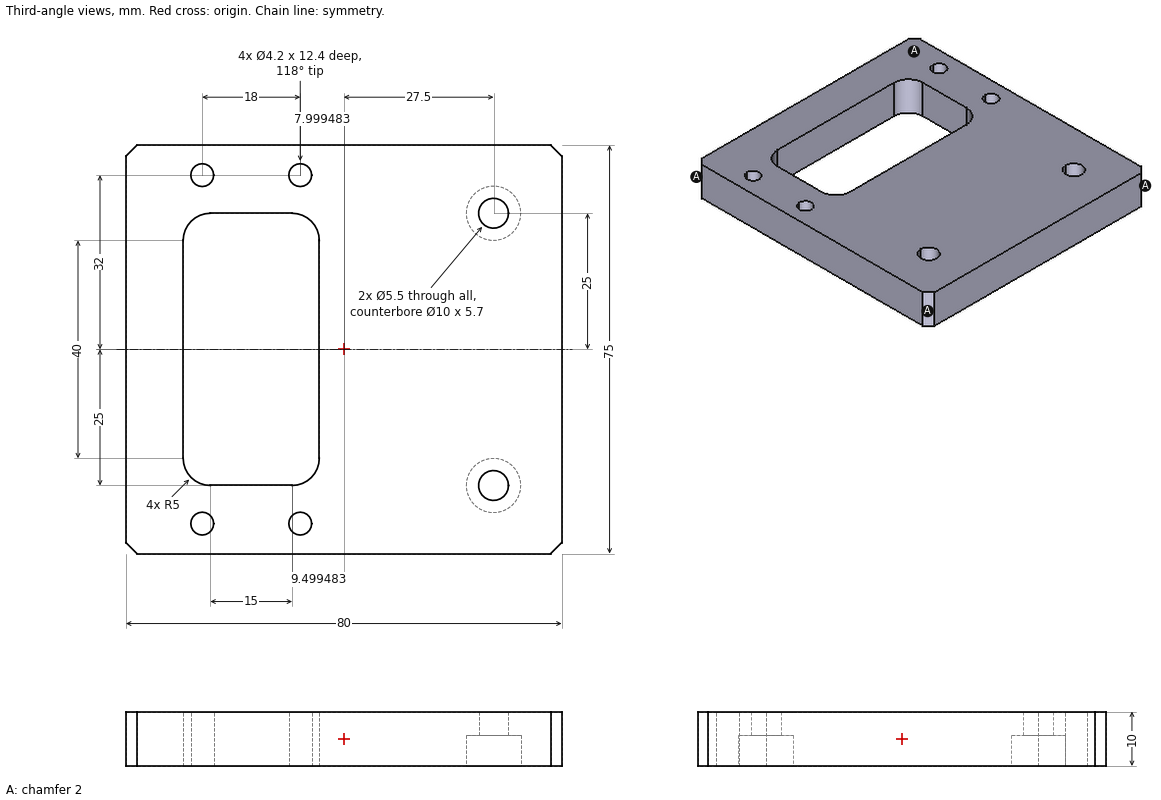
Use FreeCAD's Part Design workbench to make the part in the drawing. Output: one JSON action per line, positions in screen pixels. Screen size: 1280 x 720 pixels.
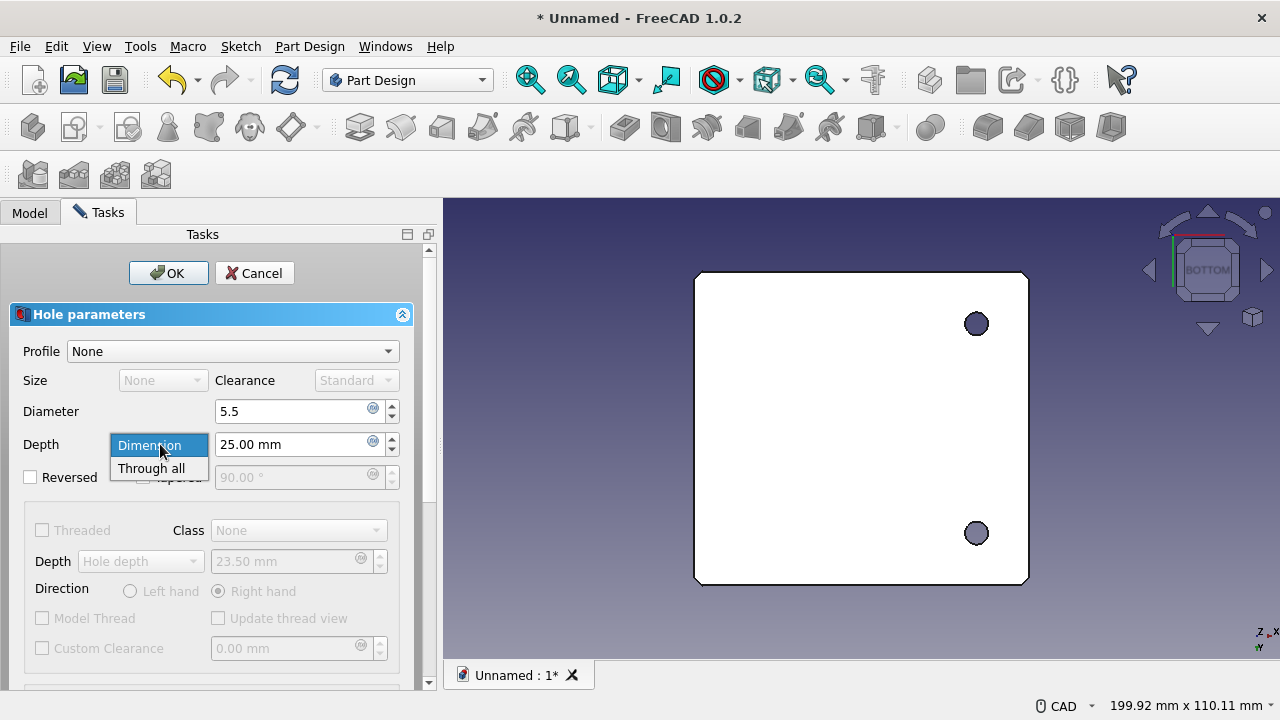
{"action": "left_click", "coordinate": [158, 468]}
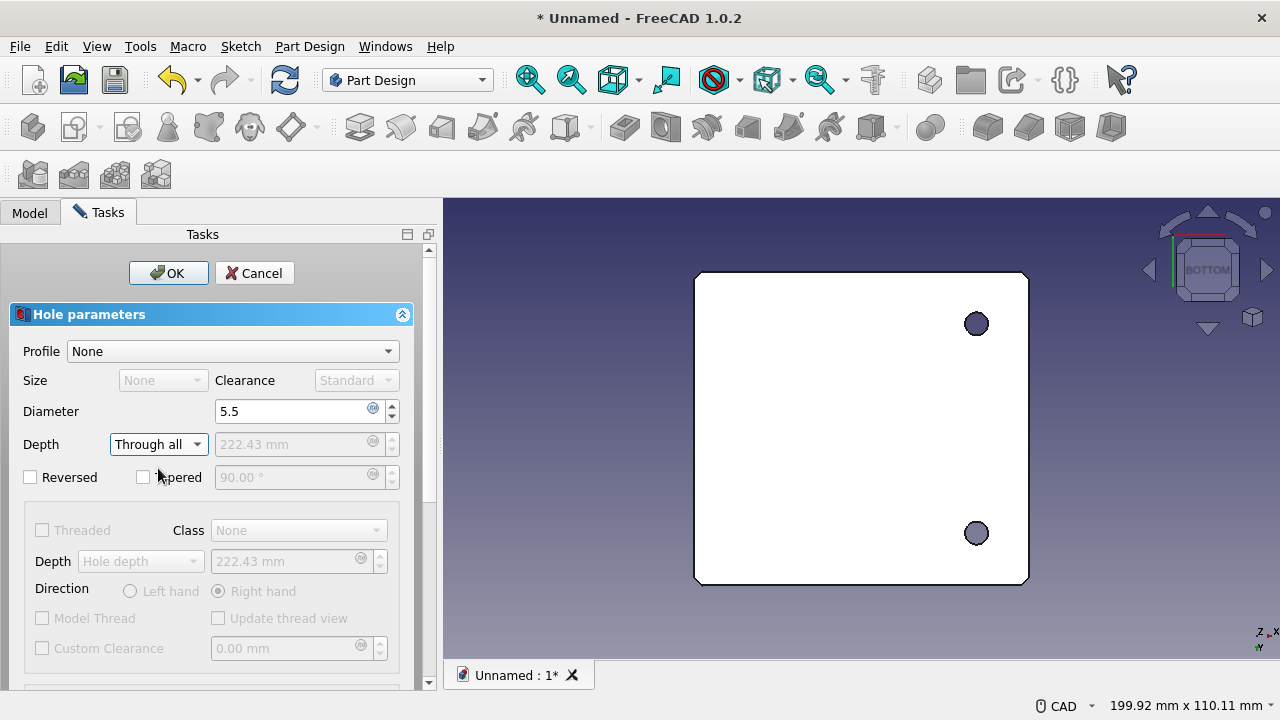
{"action": "scroll", "coordinate": [429, 467], "scroll_direction": "down", "scroll_amount": 2}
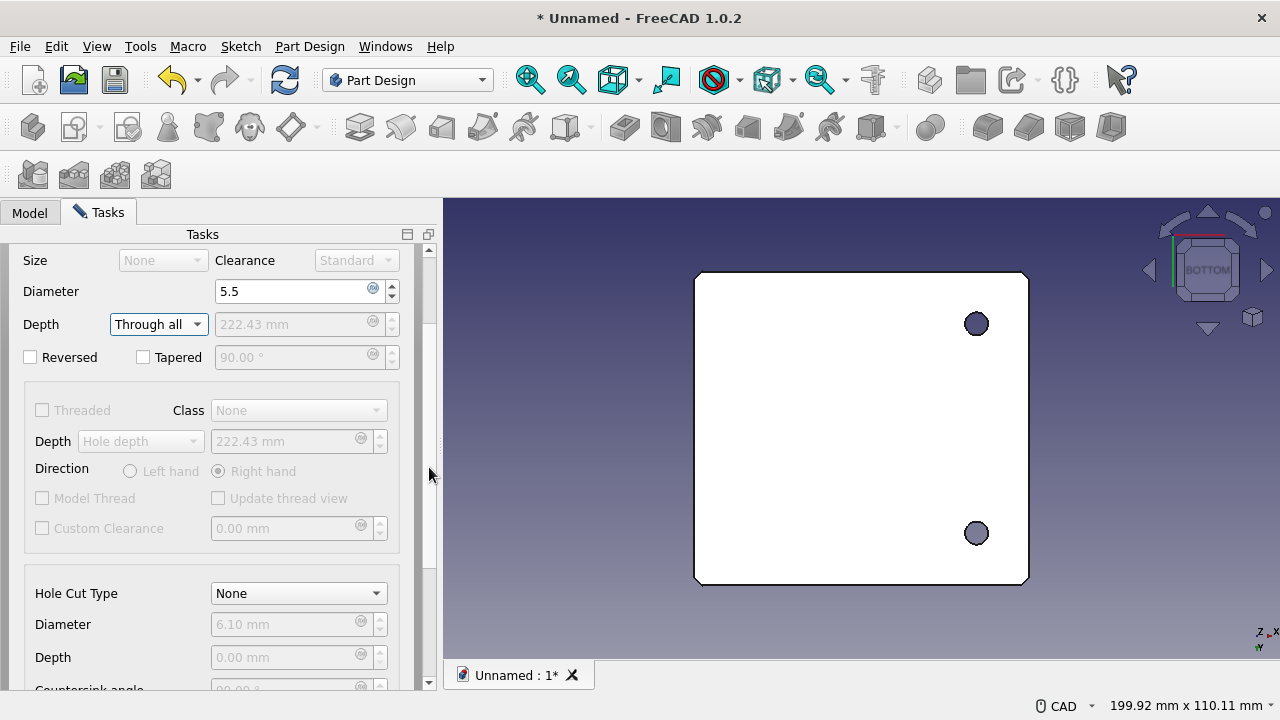
{"action": "left_click", "coordinate": [300, 594]}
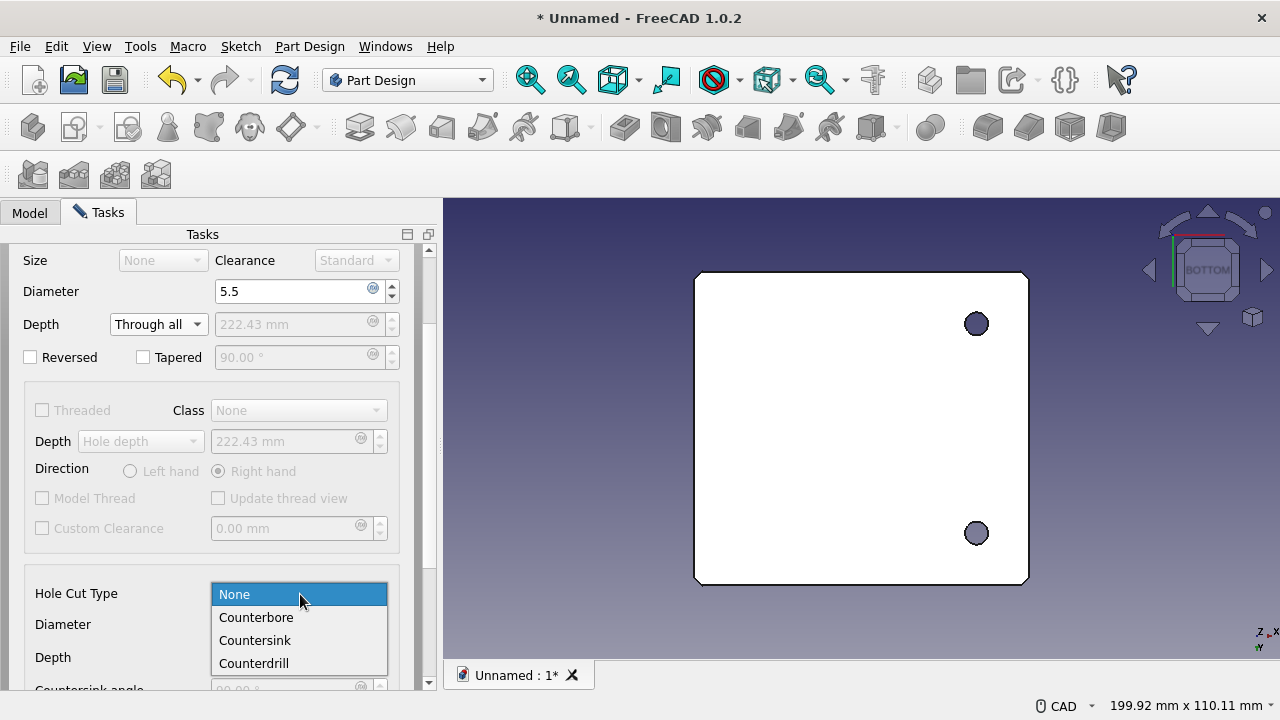
{"action": "left_click", "coordinate": [298, 618]}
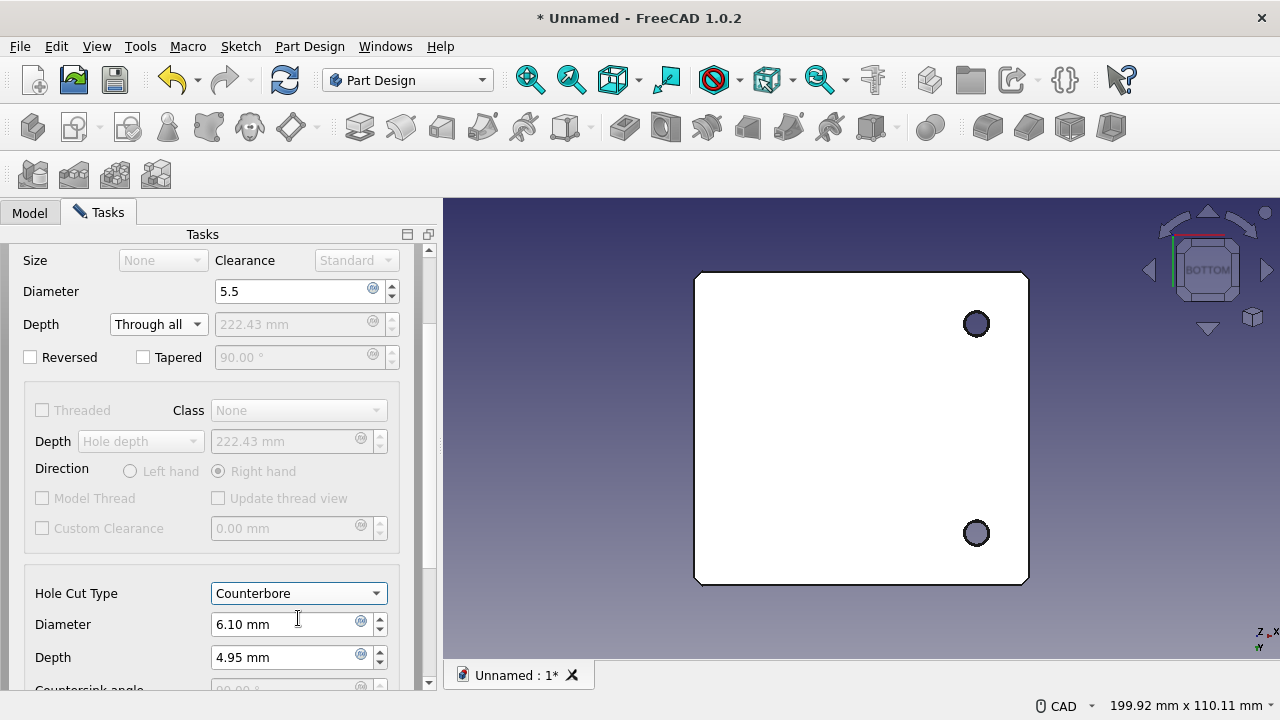
{"action": "triple_click", "coordinate": [292, 624]}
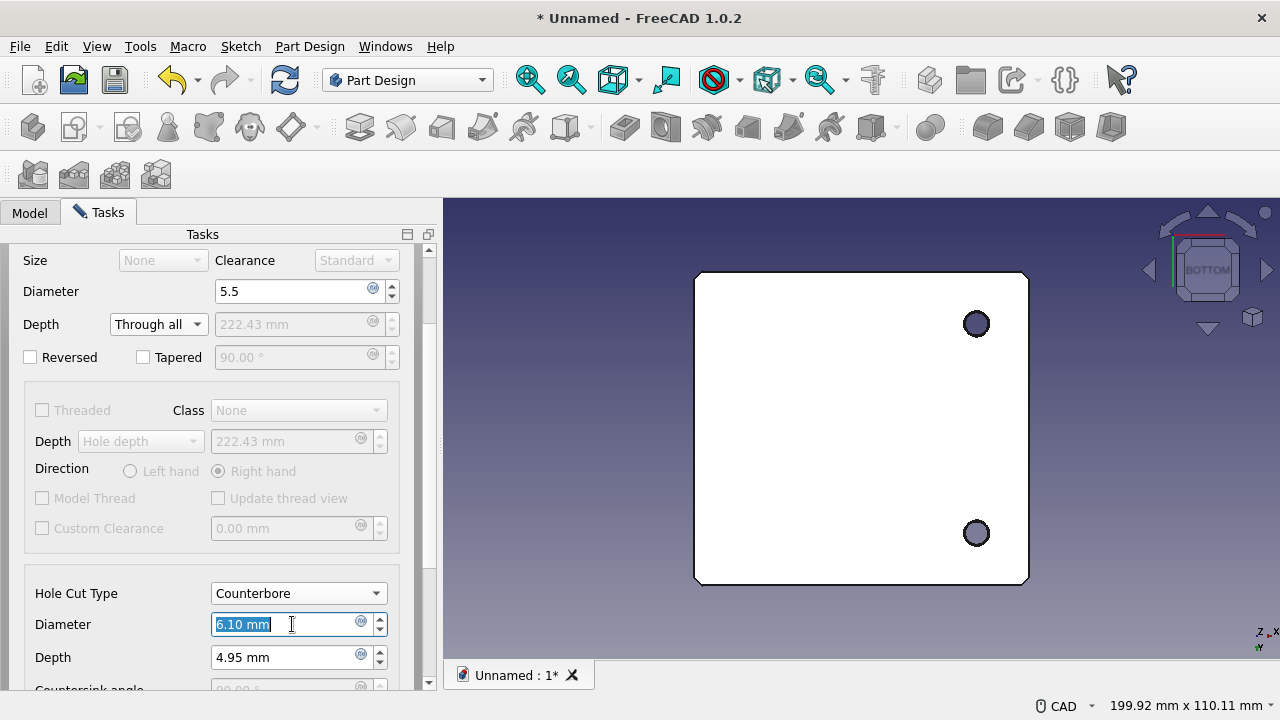
{"action": "type", "text": "10"}
{"action": "key", "text": "Tab"}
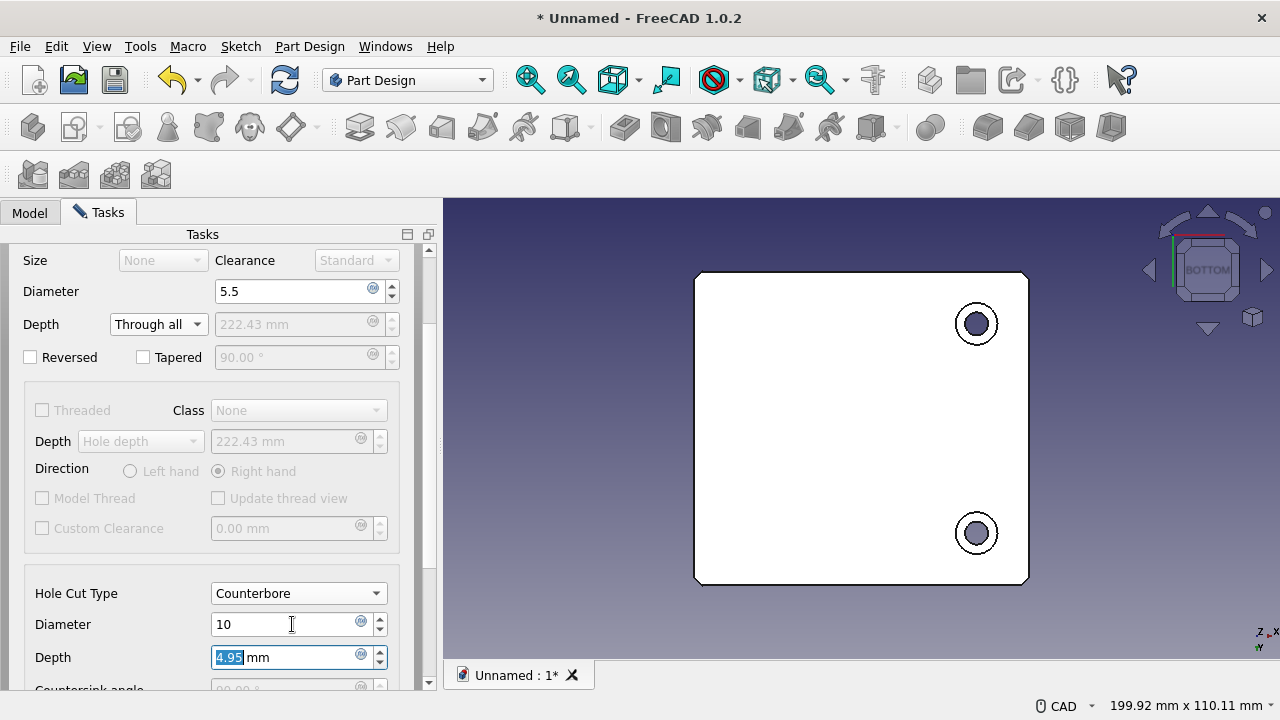
{"action": "type", "text": "5.7"}
{"action": "key", "text": "Tab"}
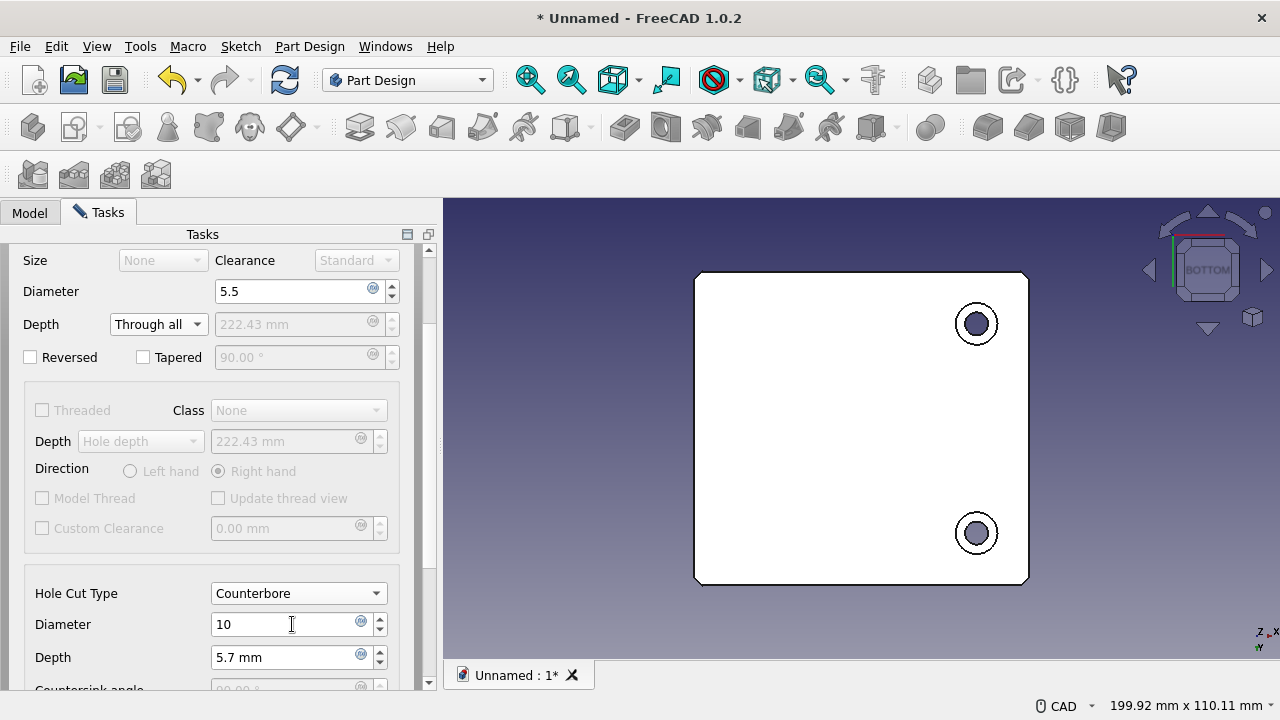
{"action": "scroll", "coordinate": [429, 467], "scroll_direction": "up", "scroll_amount": 3}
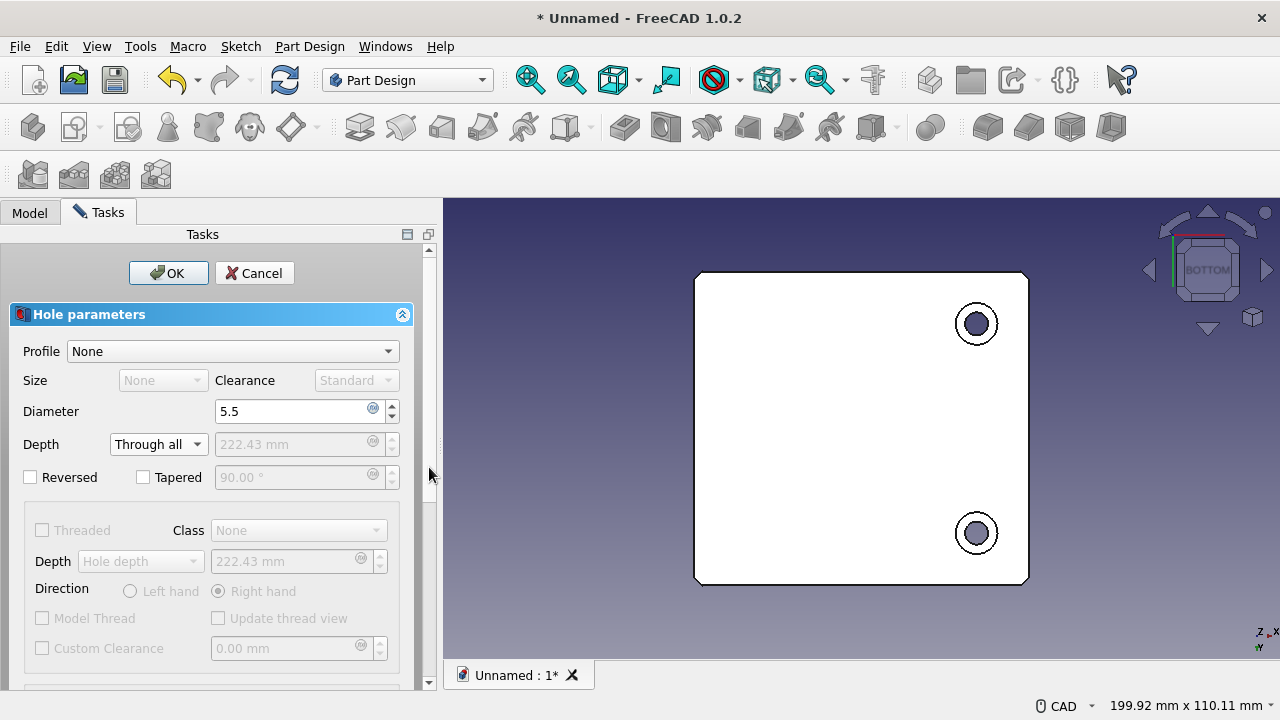
{"action": "left_click", "coordinate": [169, 273]}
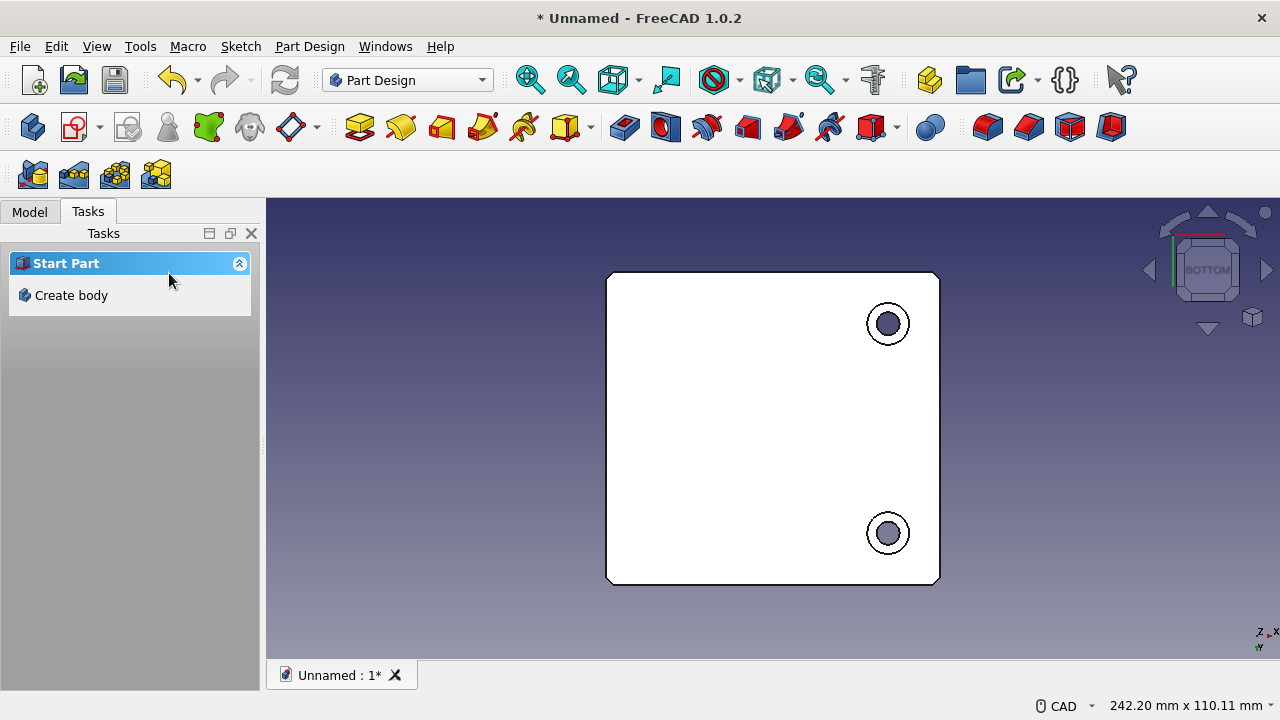
{"action": "left_click", "coordinate": [773, 428]}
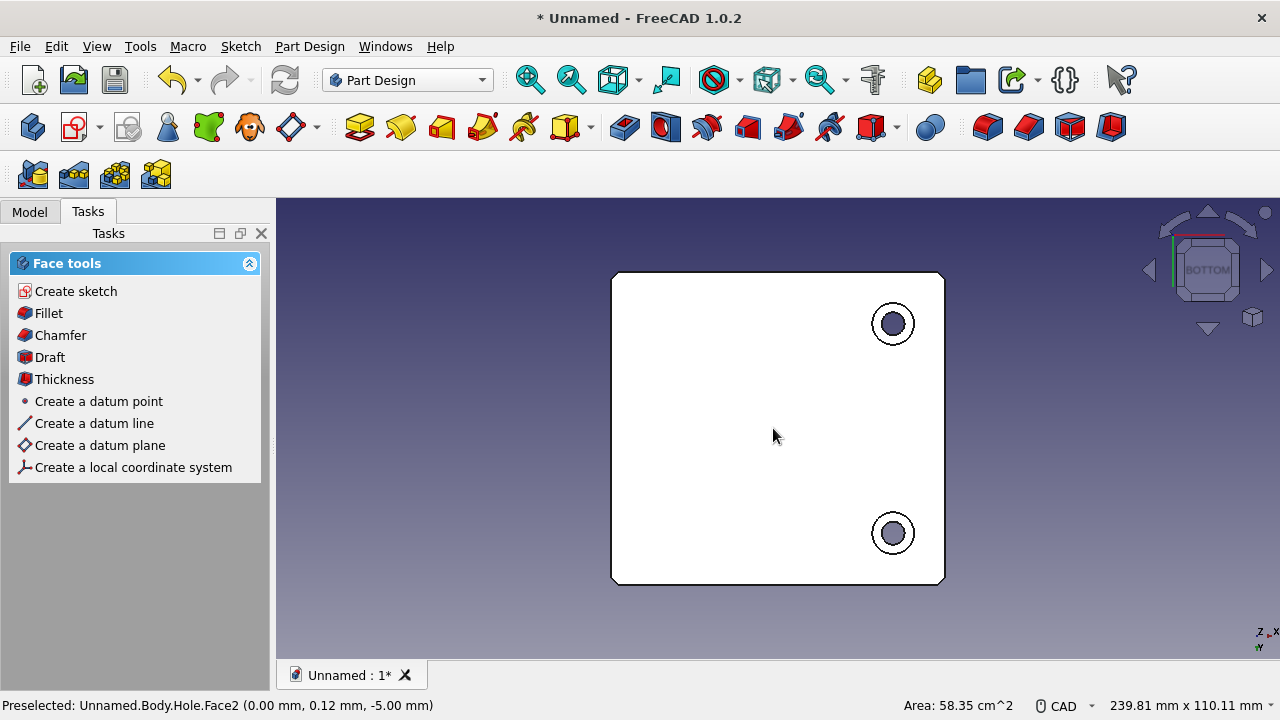
{"action": "left_click", "coordinate": [74, 128]}